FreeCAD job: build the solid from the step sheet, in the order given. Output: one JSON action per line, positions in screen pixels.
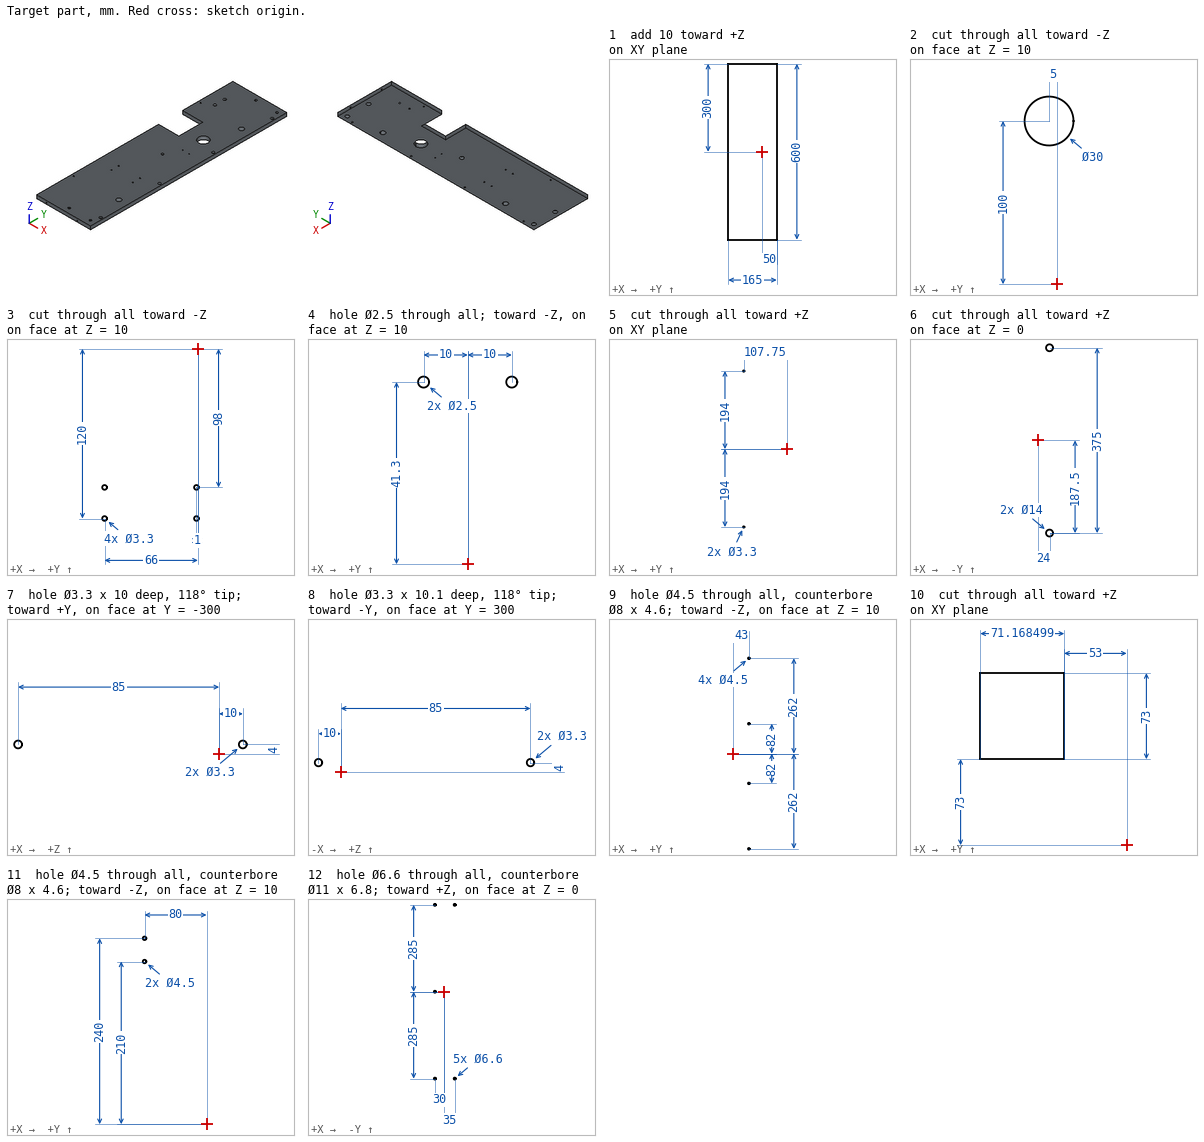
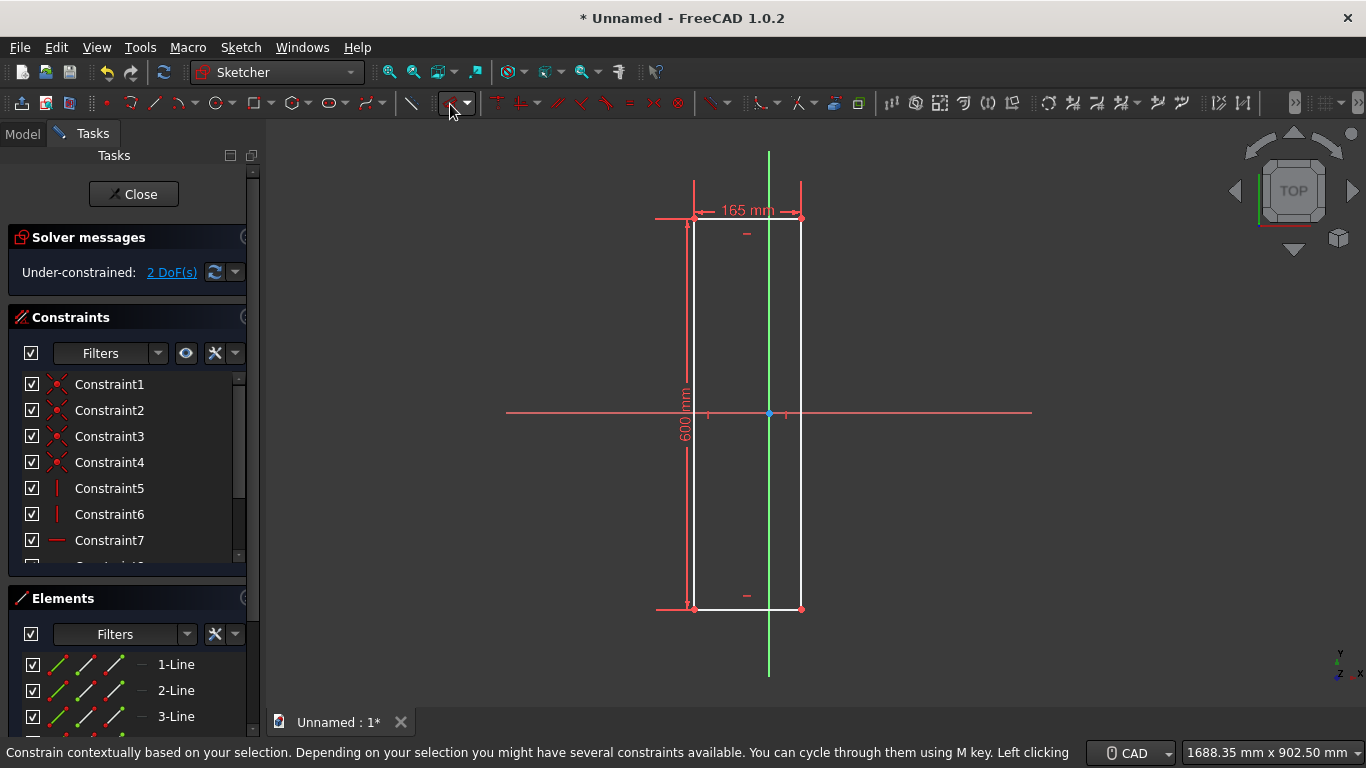
{"action": "left_click", "coordinate": [802, 610]}
{"action": "left_click", "coordinate": [785, 644]}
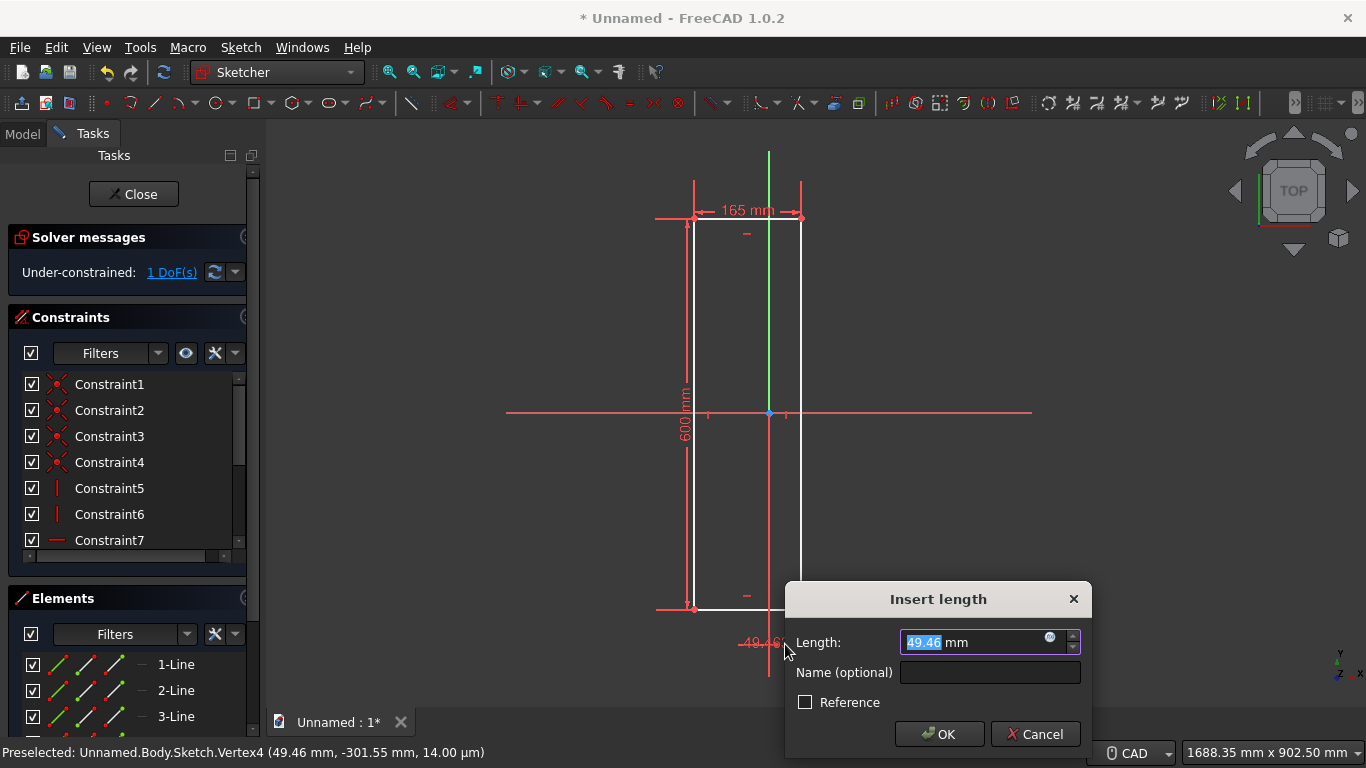
{"action": "type", "text": "50"}
{"action": "key", "text": "Return"}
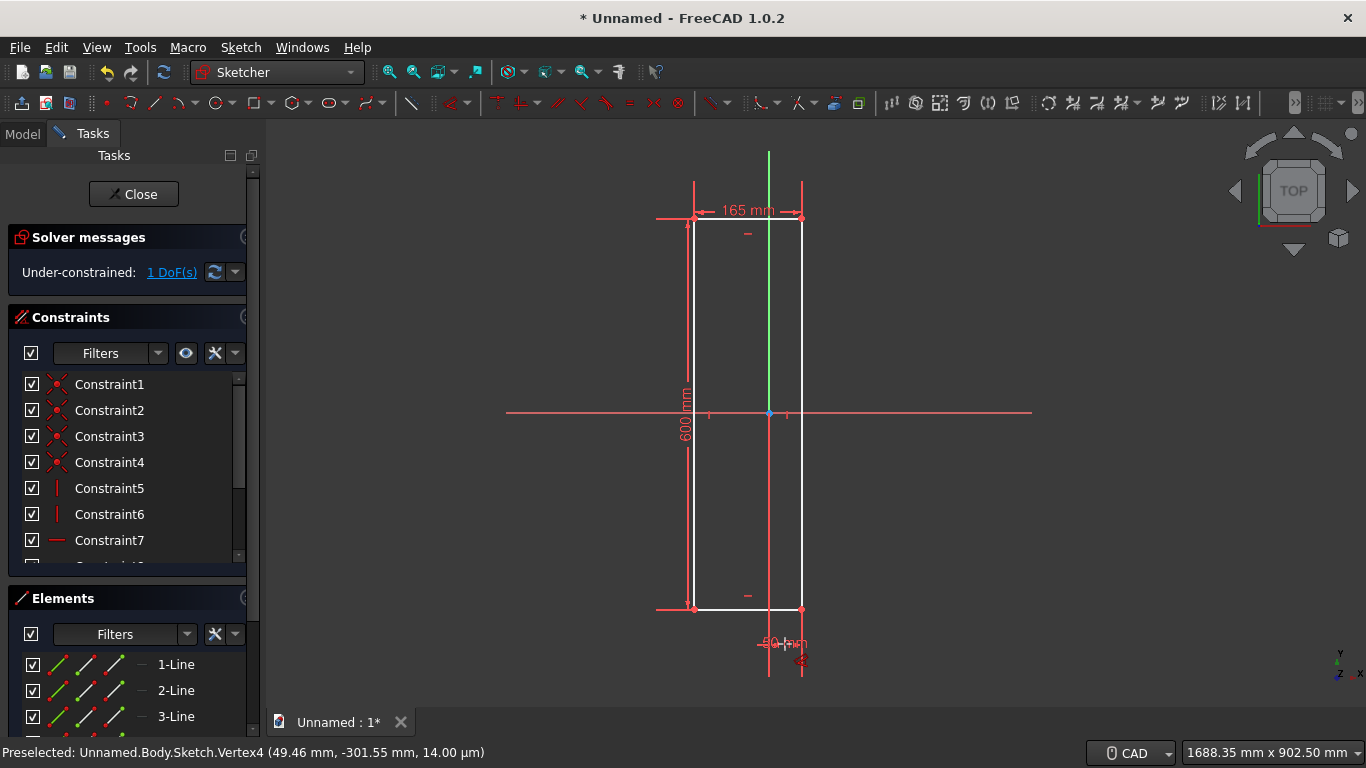
{"action": "left_click", "coordinate": [694, 219]}
{"action": "left_click", "coordinate": [660, 316]}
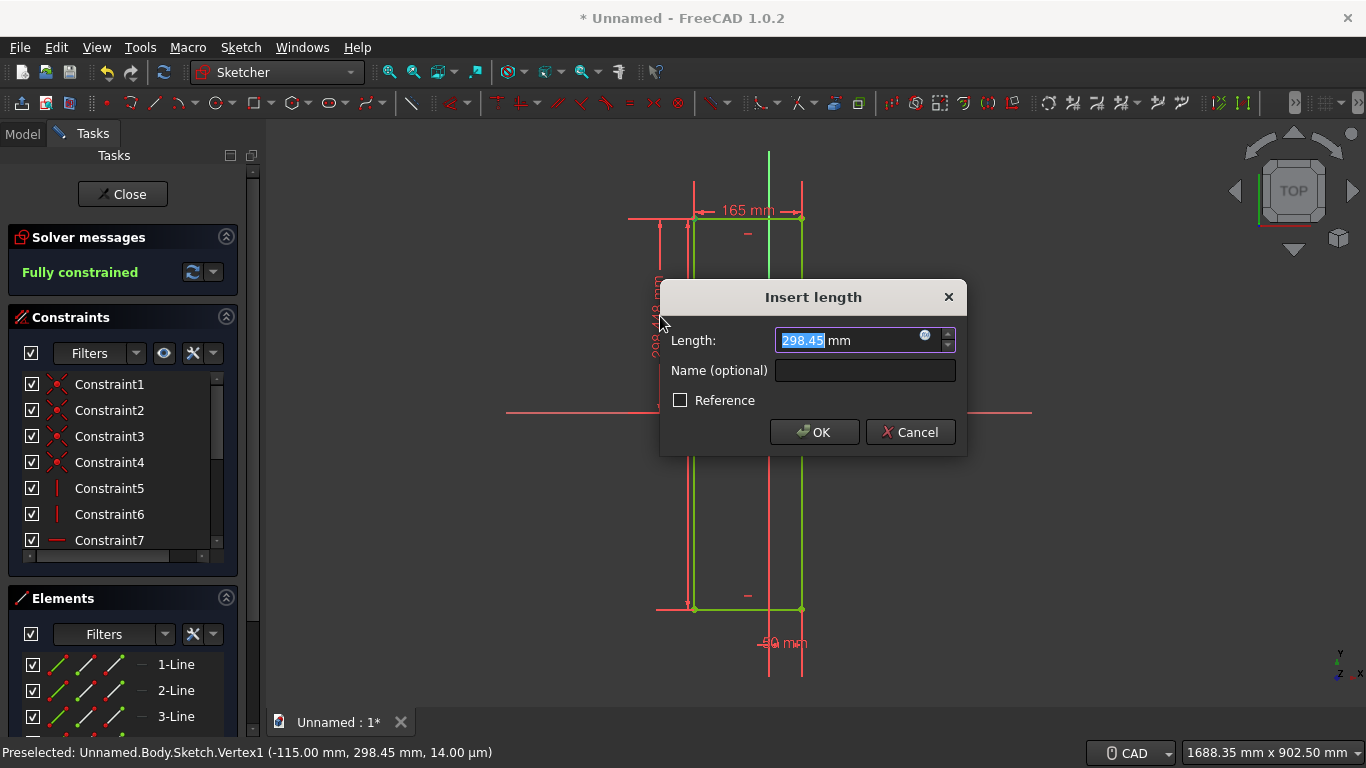
{"action": "type", "text": "300"}
{"action": "key", "text": "Return"}
{"action": "key", "text": "Escape"}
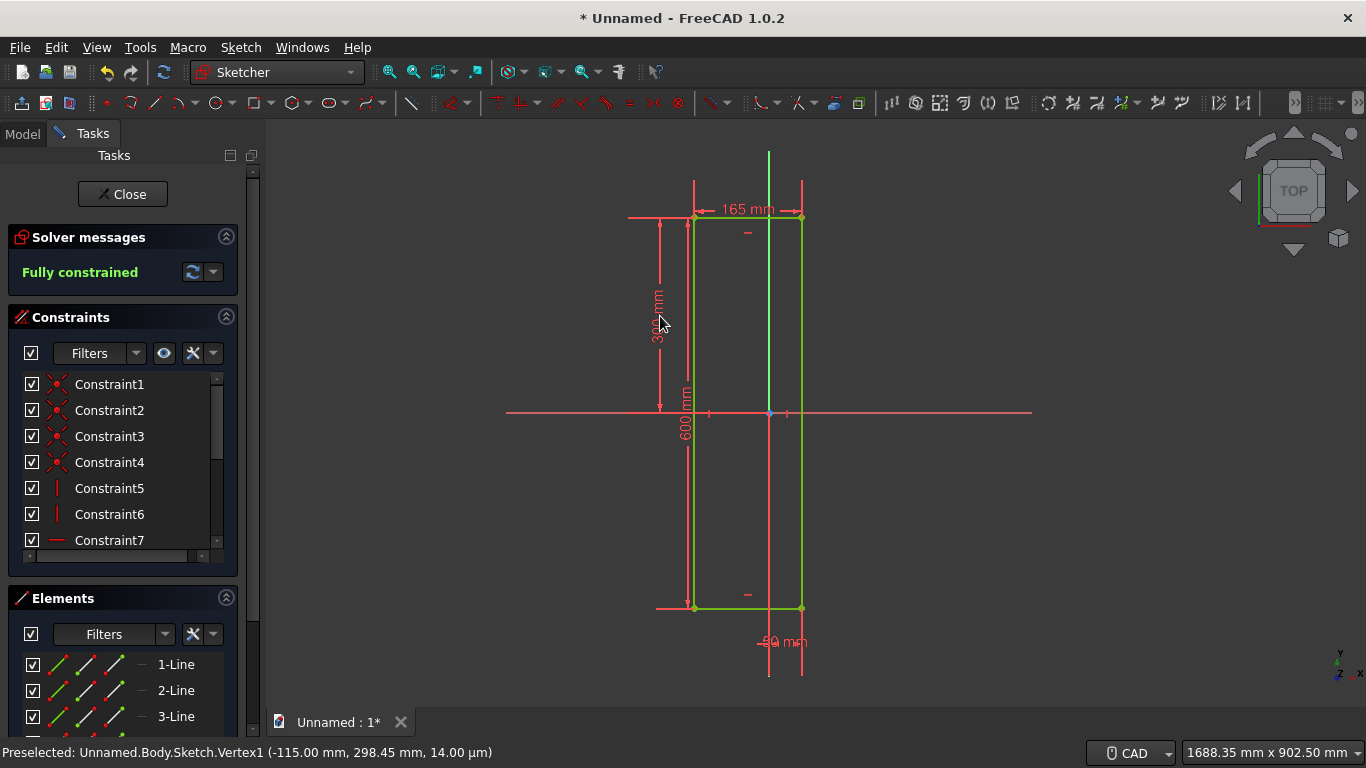
{"action": "left_click", "coordinate": [123, 194]}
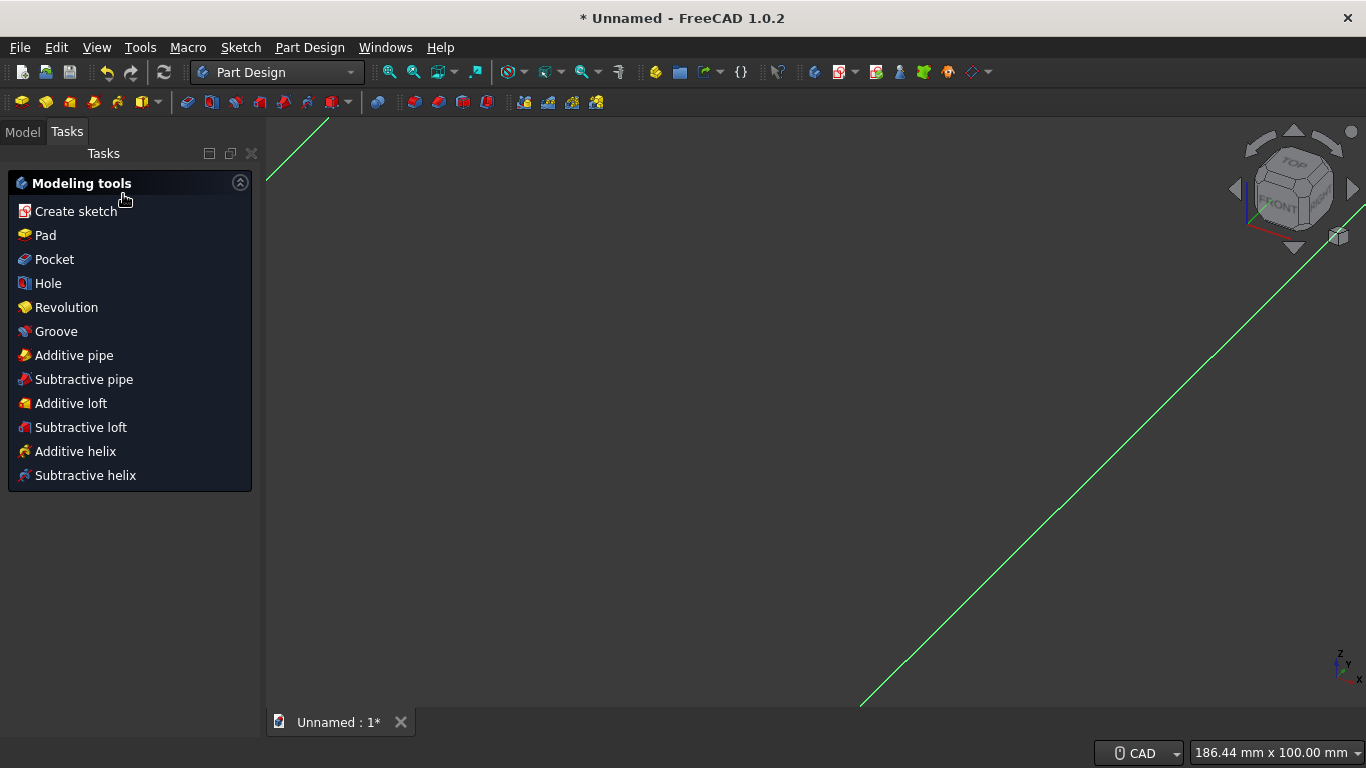
{"action": "left_click", "coordinate": [22, 102]}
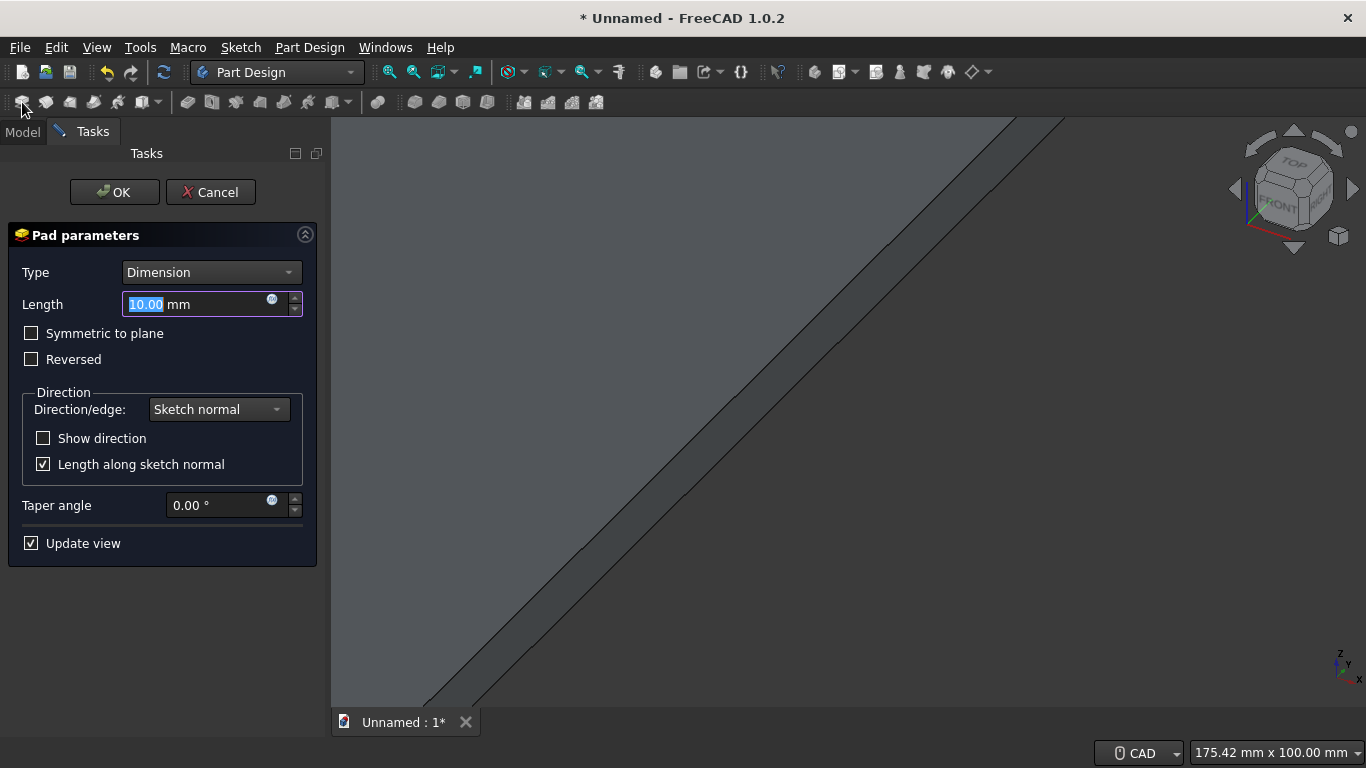
{"action": "type", "text": "10"}
{"action": "key", "text": "Tab"}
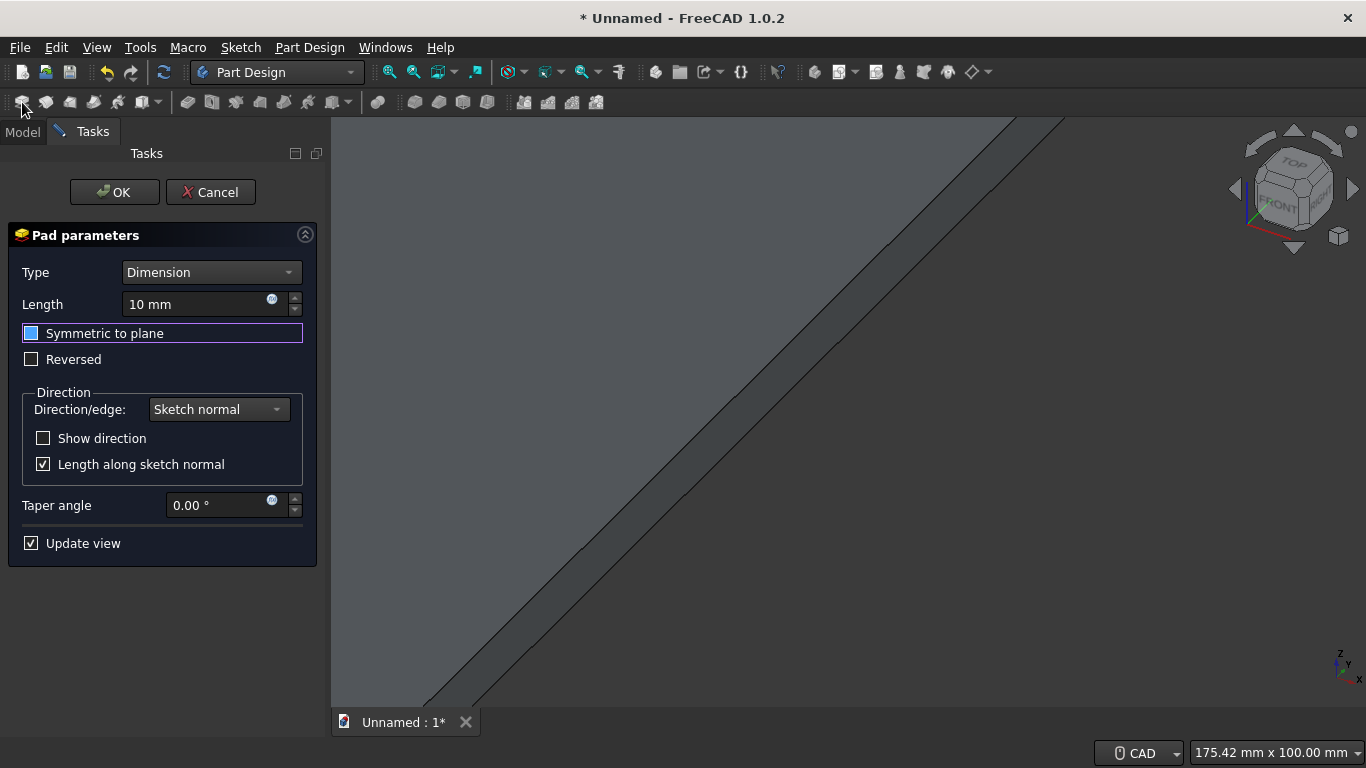
{"action": "left_click", "coordinate": [115, 192]}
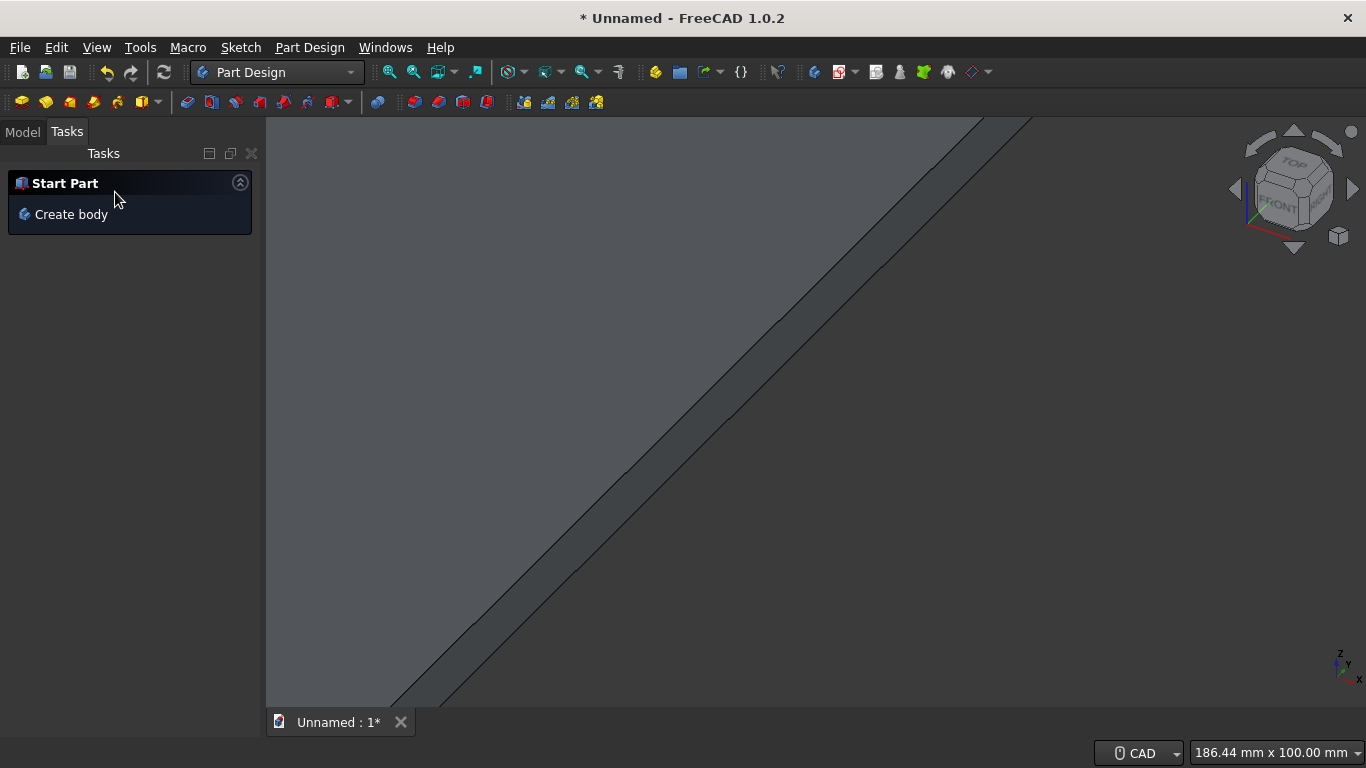
{"action": "key", "text": "v f"}